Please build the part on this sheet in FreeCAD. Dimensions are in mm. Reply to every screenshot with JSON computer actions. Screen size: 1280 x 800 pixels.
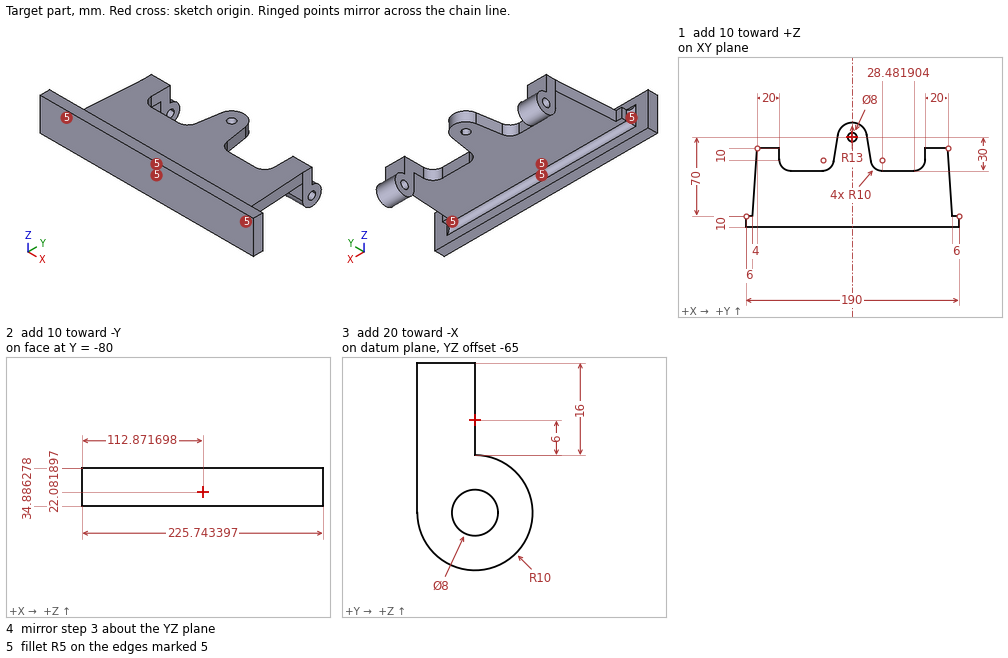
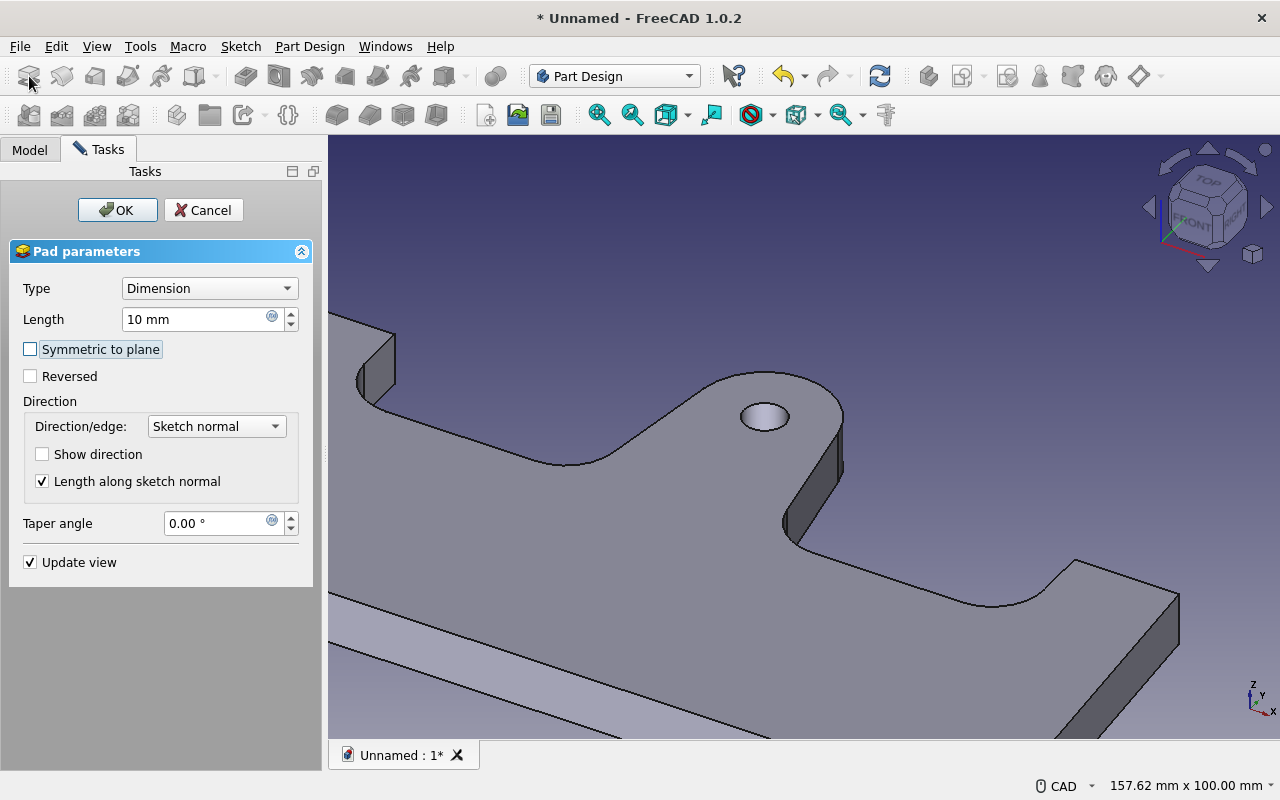
{"action": "left_click", "coordinate": [118, 210]}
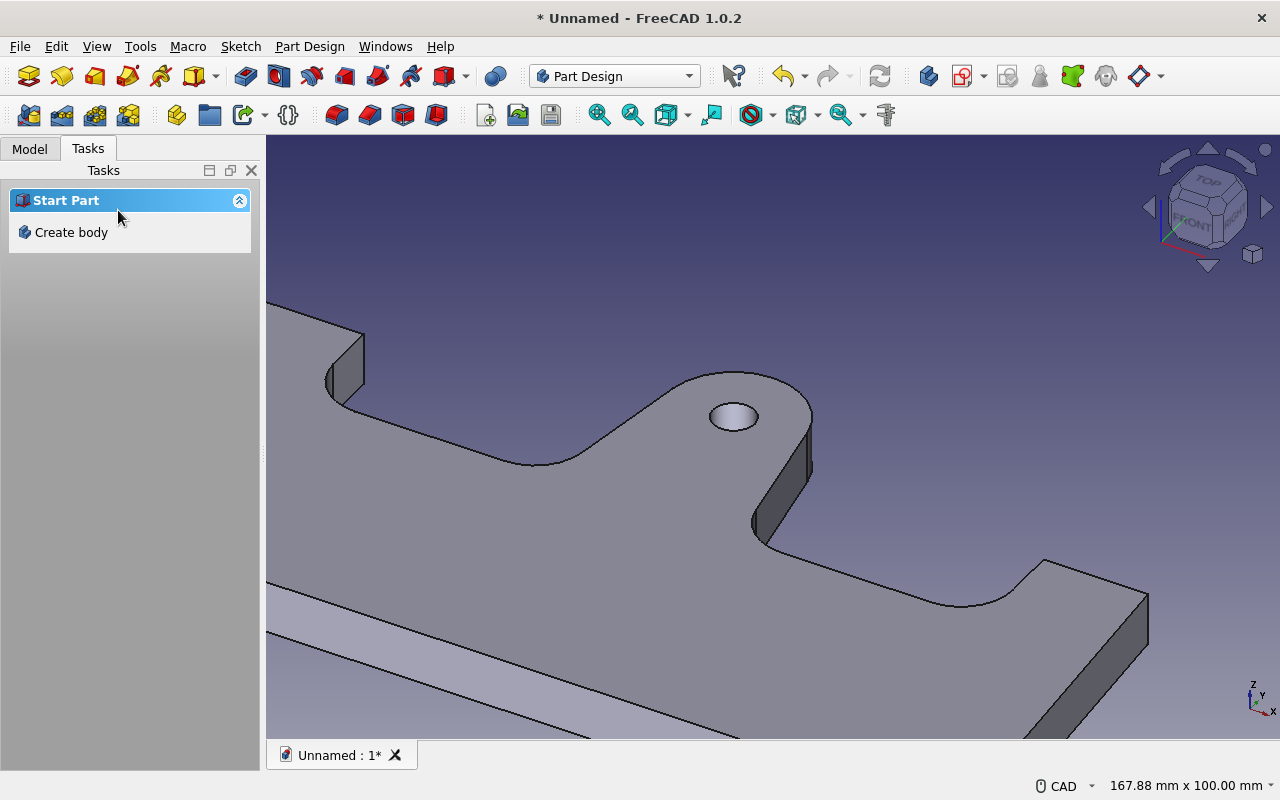
{"action": "left_click", "coordinate": [600, 116]}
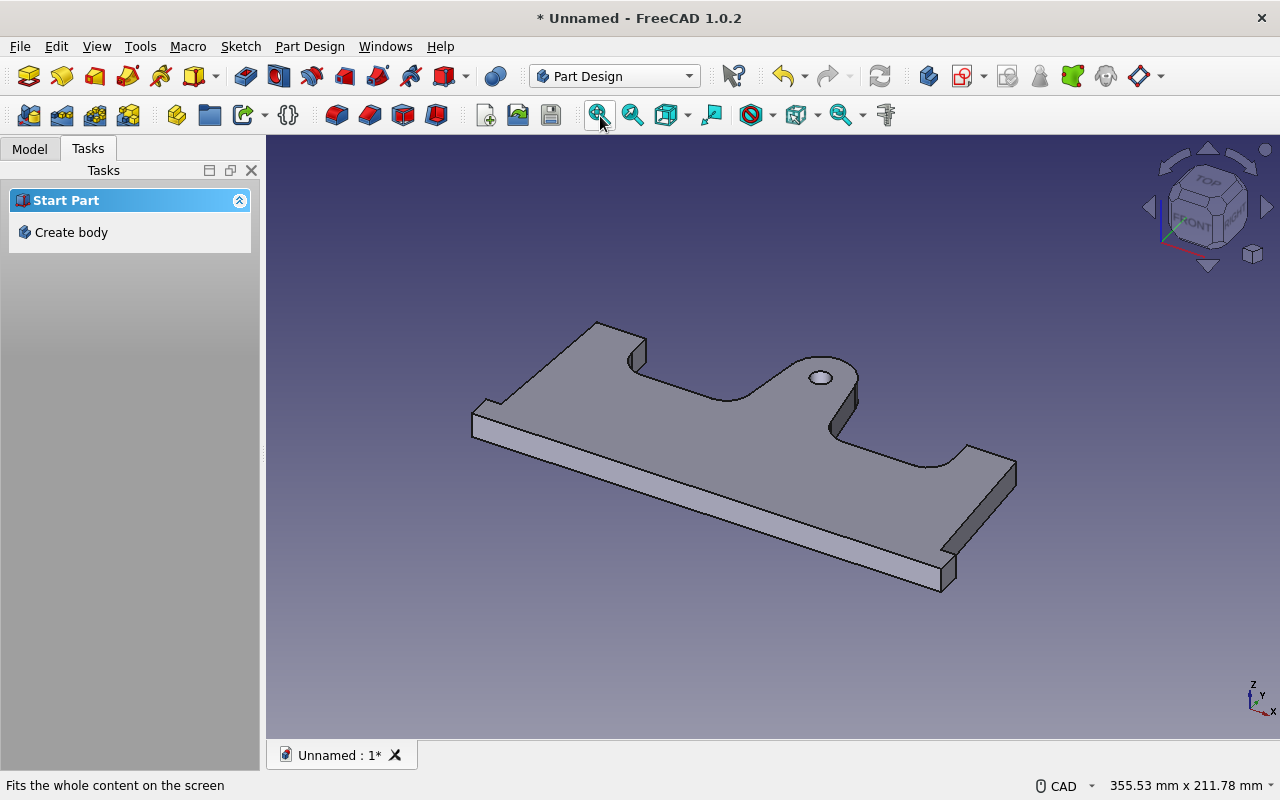
{"action": "left_click", "coordinate": [908, 568]}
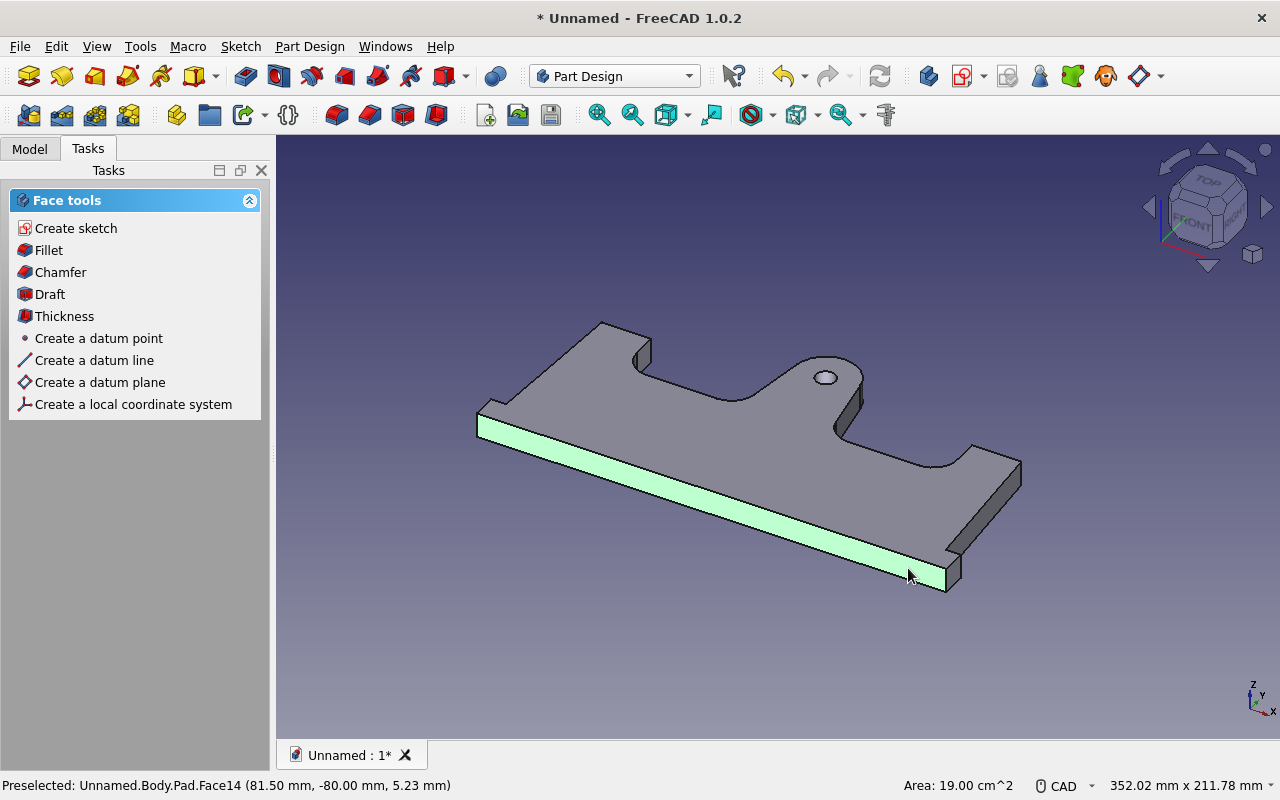
{"action": "left_click", "coordinate": [962, 76]}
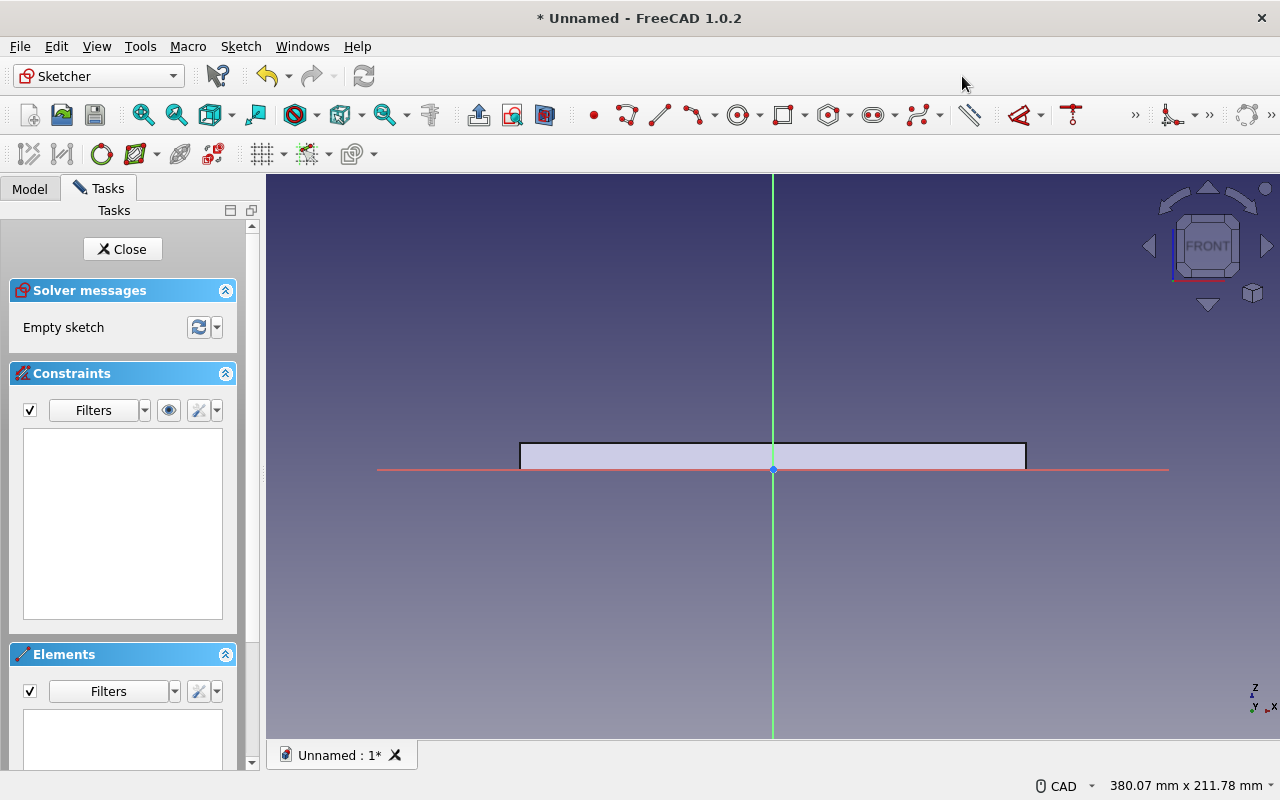
{"action": "left_click", "coordinate": [782, 116]}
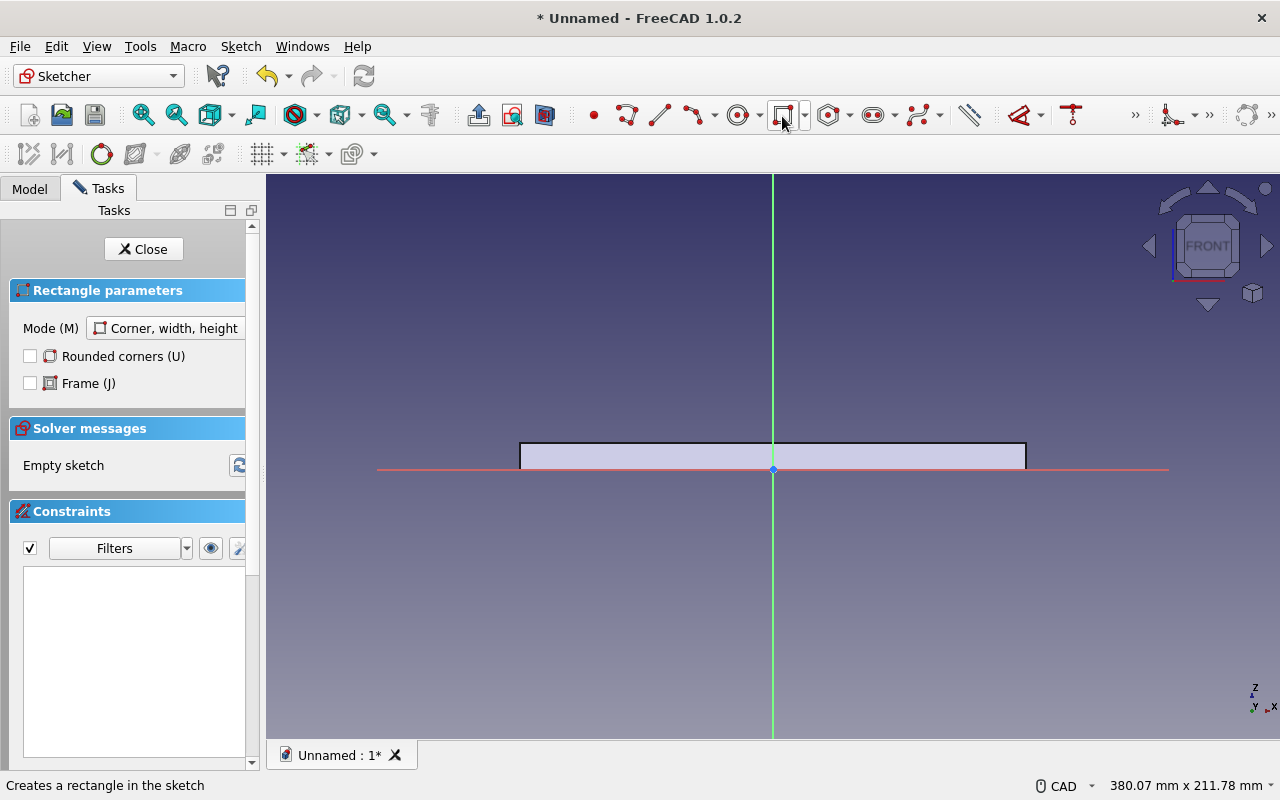
{"action": "left_click", "coordinate": [472, 411]}
{"action": "left_click", "coordinate": [1074, 504]}
{"action": "key", "text": "Escape"}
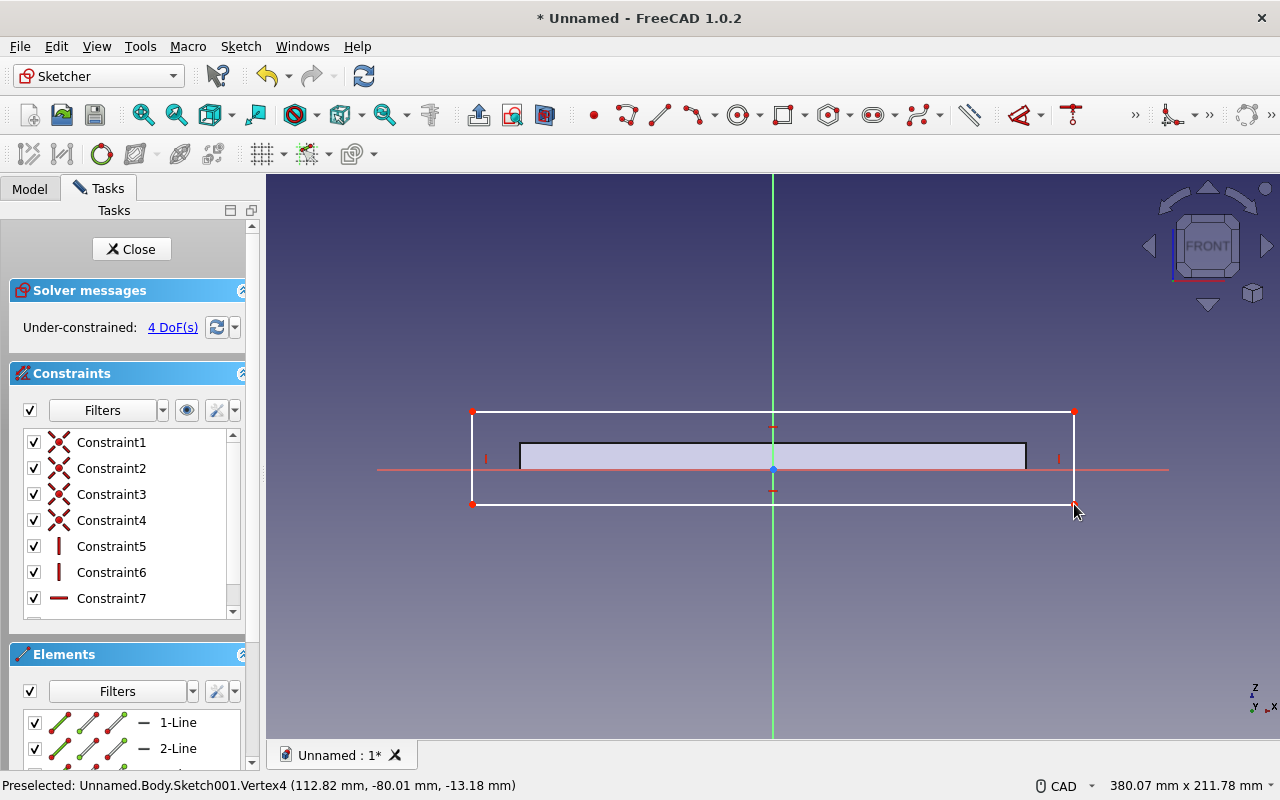
{"action": "left_click", "coordinate": [1018, 116]}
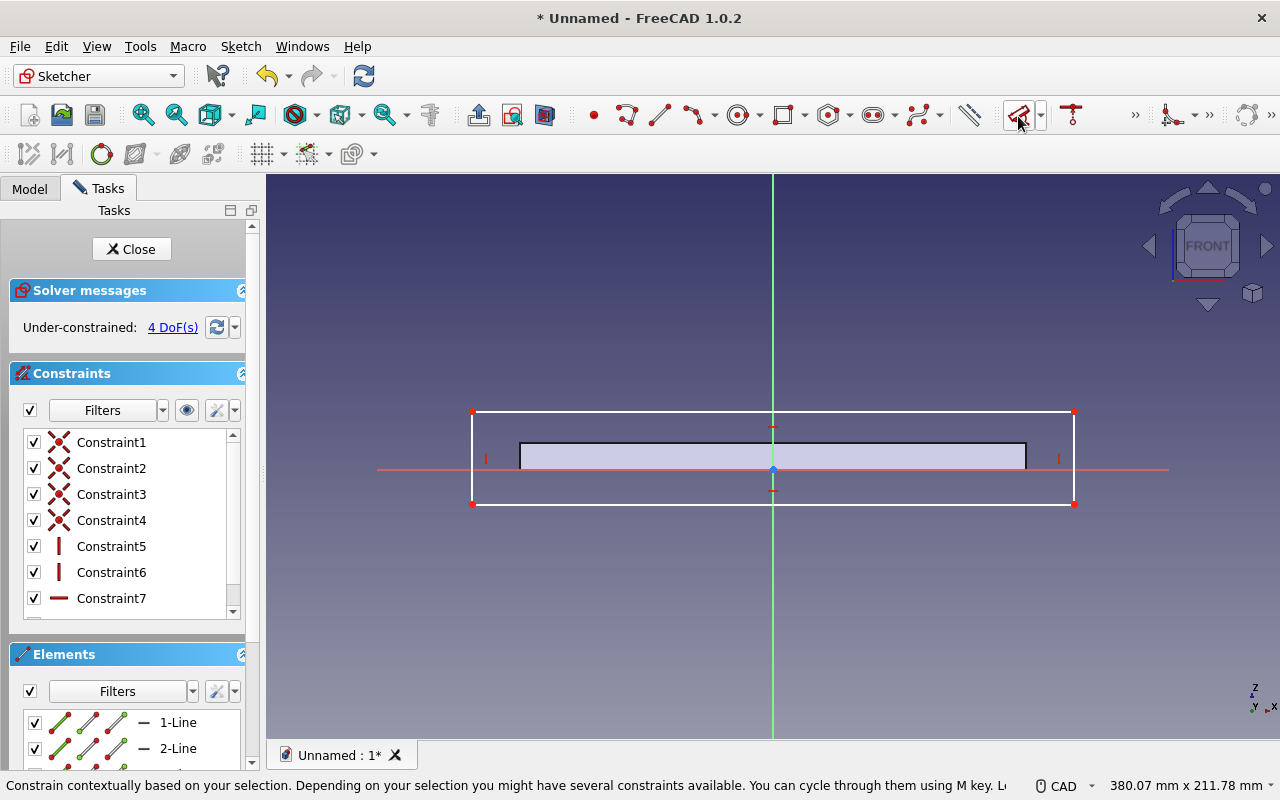
{"action": "left_click", "coordinate": [472, 440]}
{"action": "left_click", "coordinate": [438, 437]}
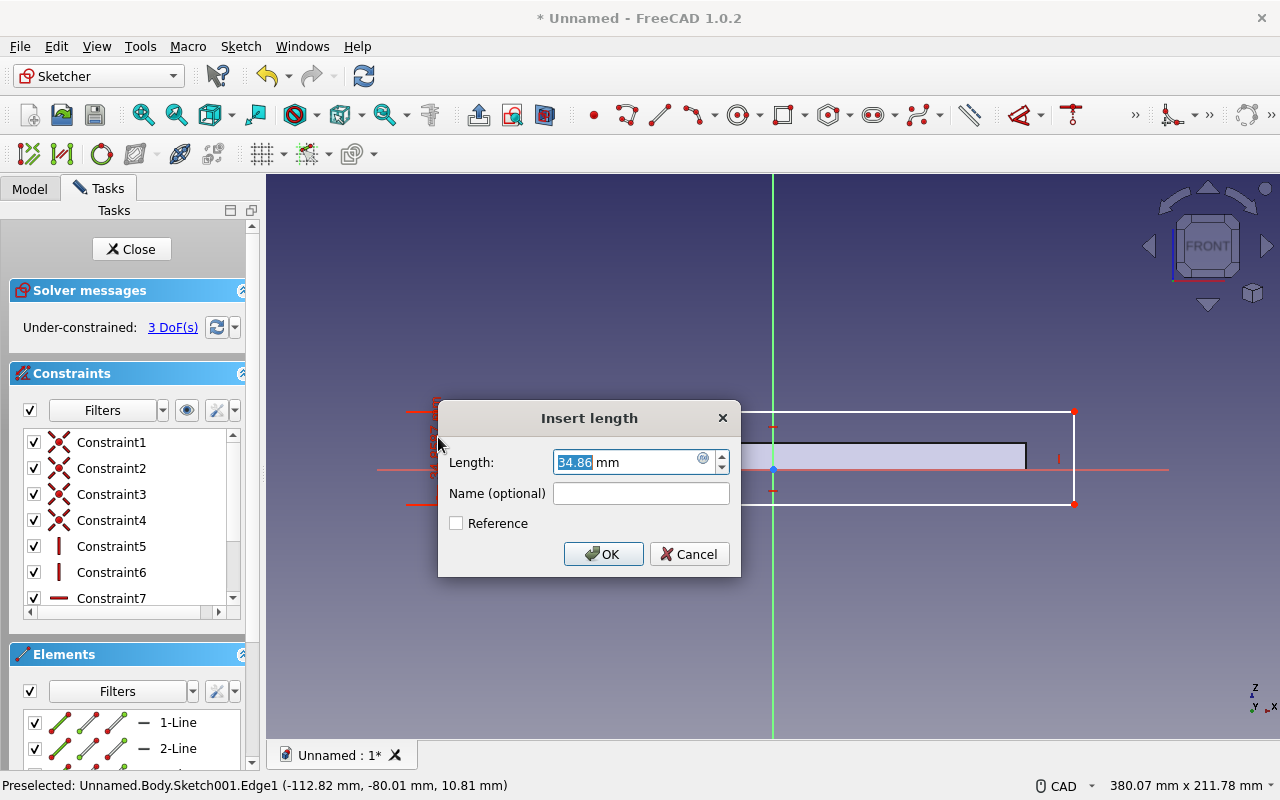
{"action": "type", "text": "34.886278"}
{"action": "key", "text": "Return"}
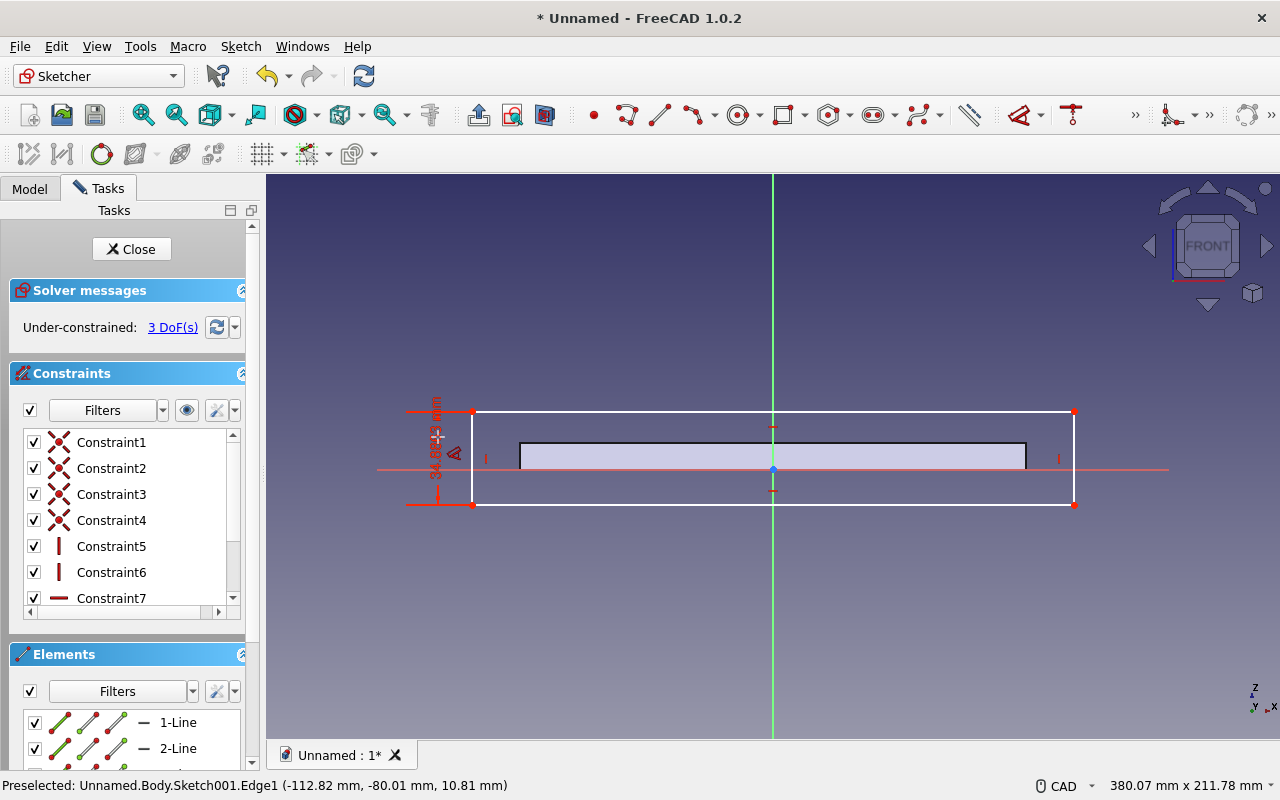
{"action": "left_click", "coordinate": [653, 505]}
{"action": "left_click", "coordinate": [635, 539]}